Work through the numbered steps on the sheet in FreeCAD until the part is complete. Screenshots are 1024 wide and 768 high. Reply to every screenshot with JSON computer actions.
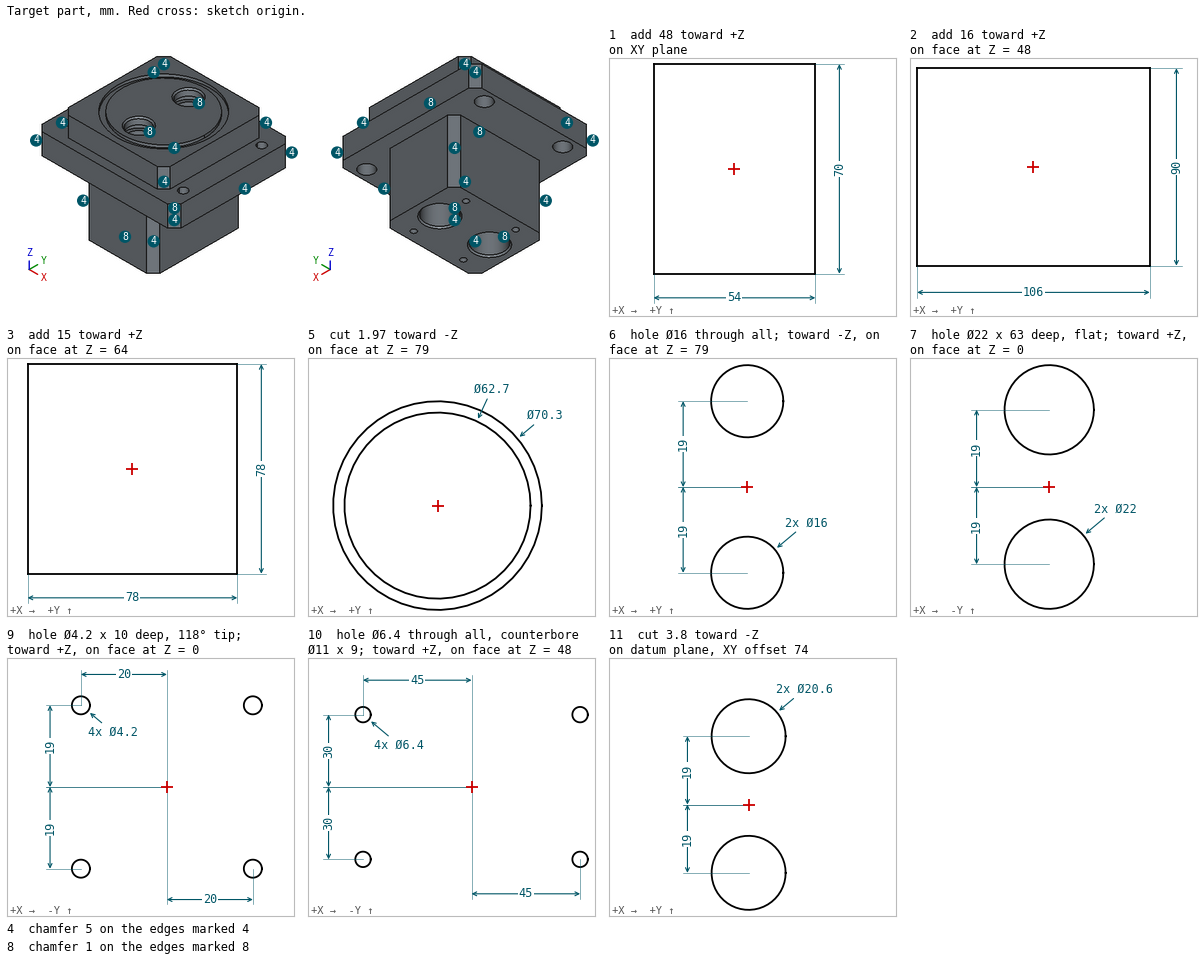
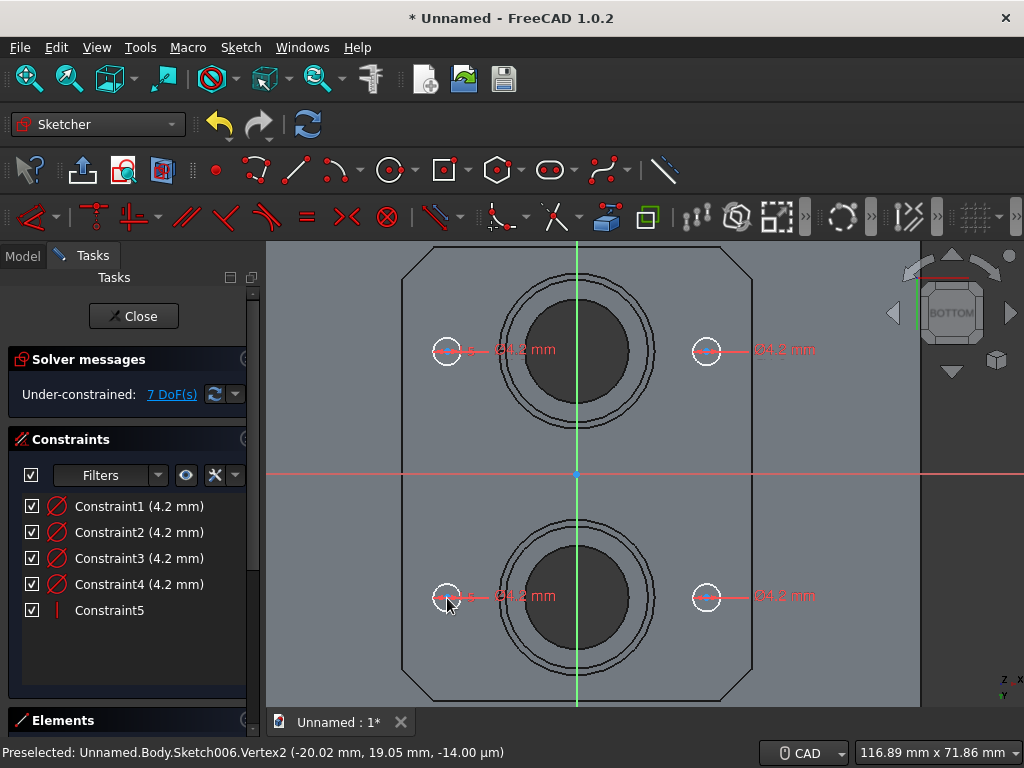
{"action": "left_click", "coordinate": [447, 598]}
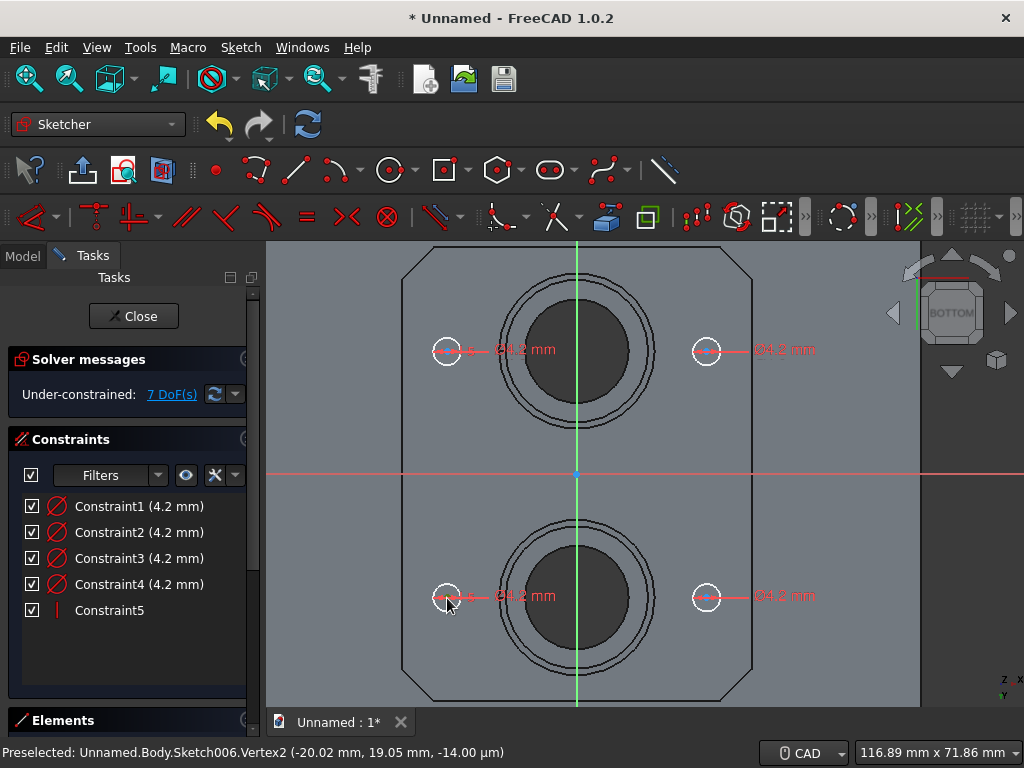
{"action": "left_click", "coordinate": [707, 598]}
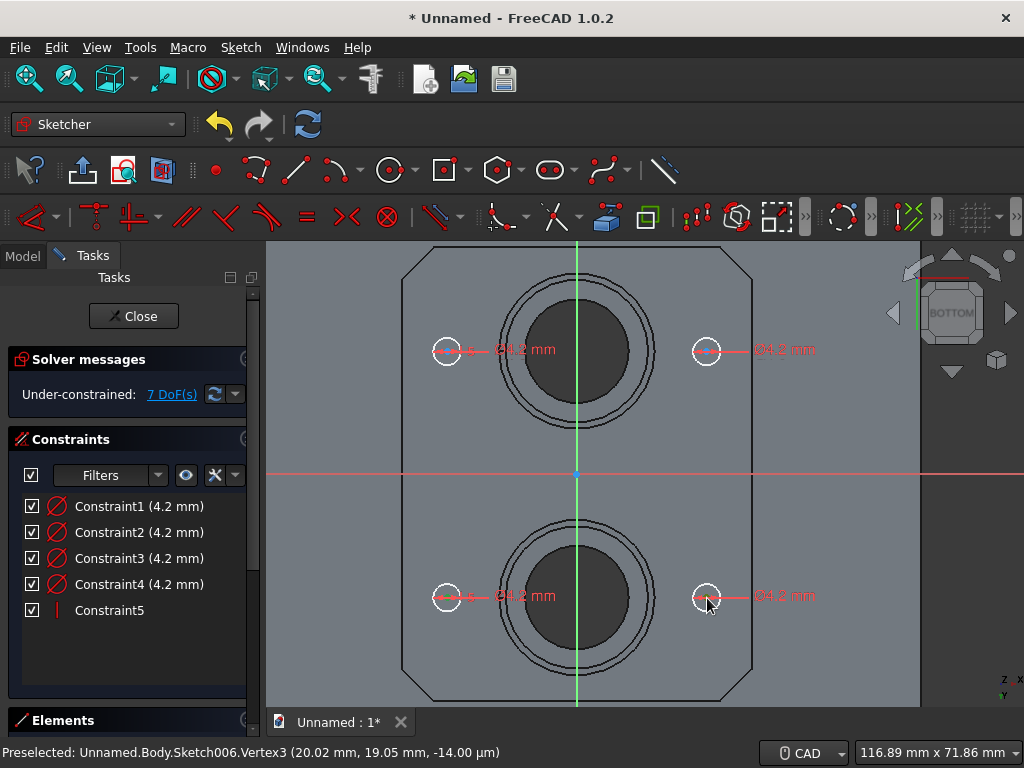
{"action": "key", "text": "h"}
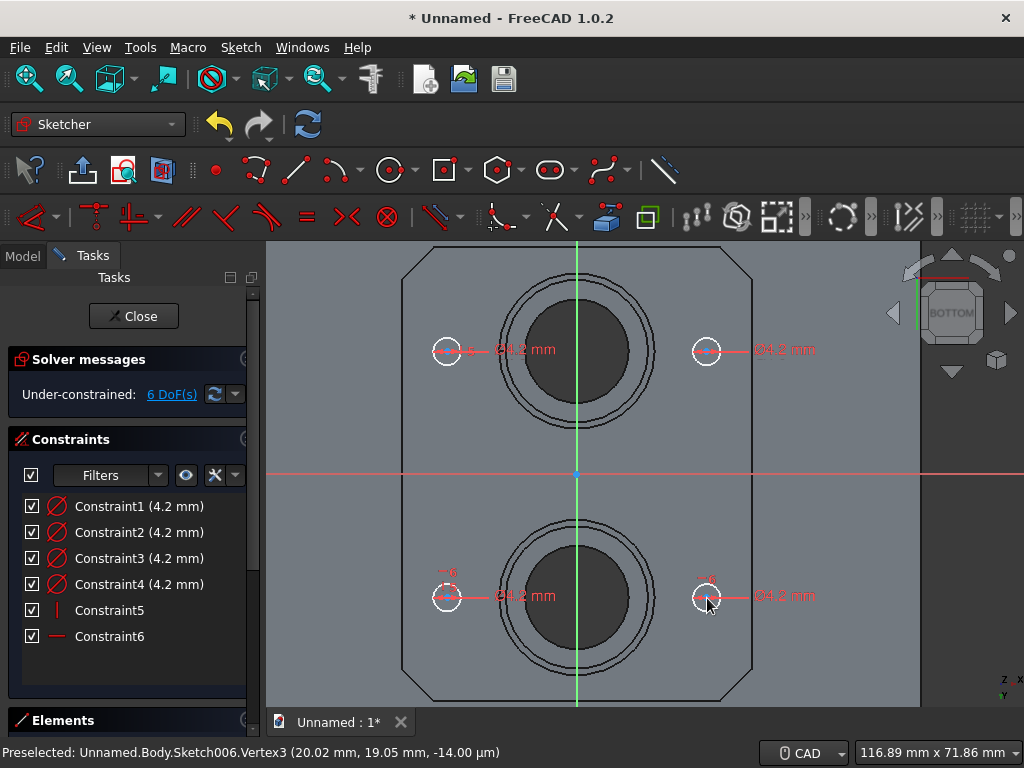
{"action": "left_click", "coordinate": [707, 598]}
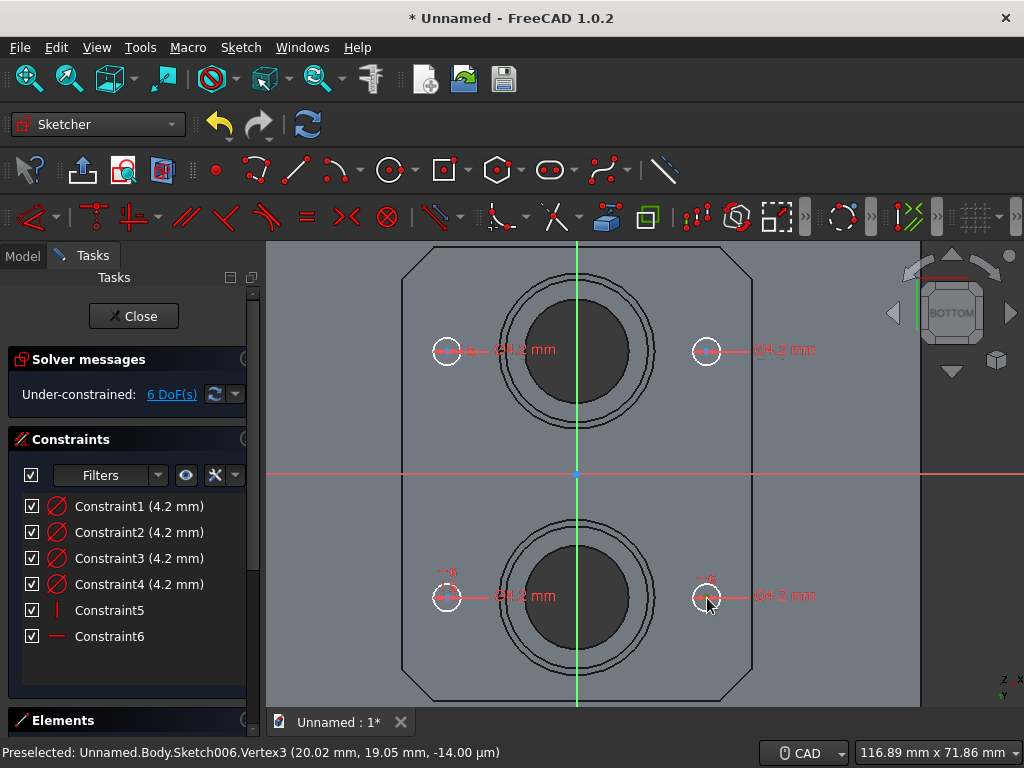
{"action": "left_click", "coordinate": [707, 352]}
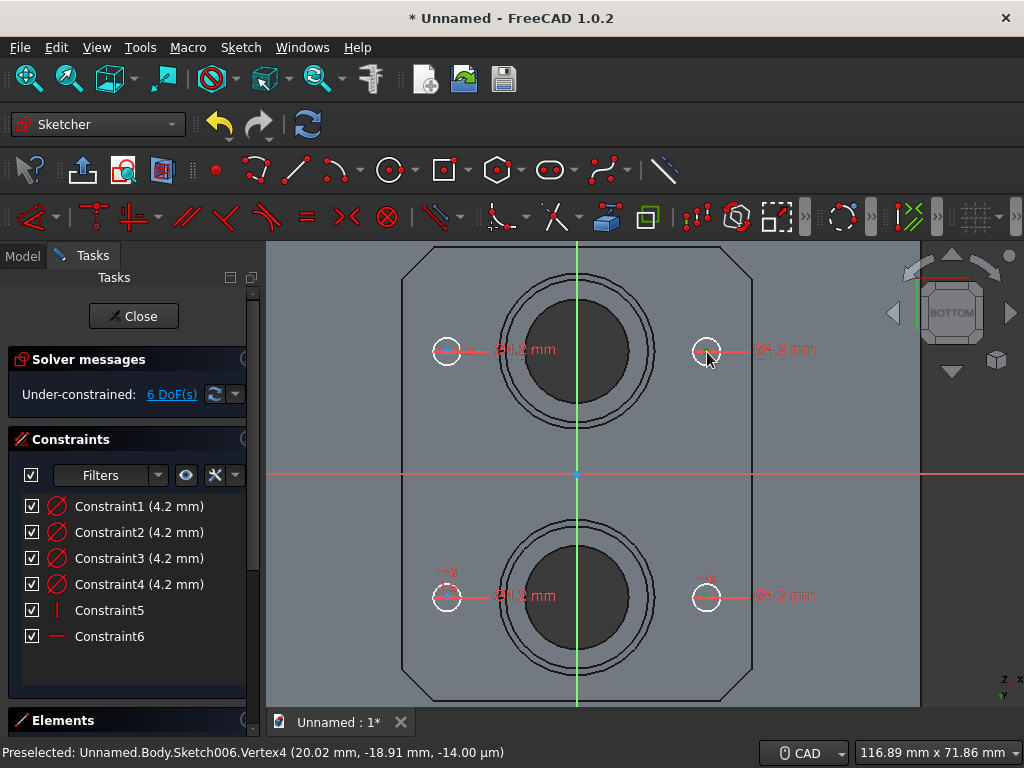
{"action": "key", "text": "v"}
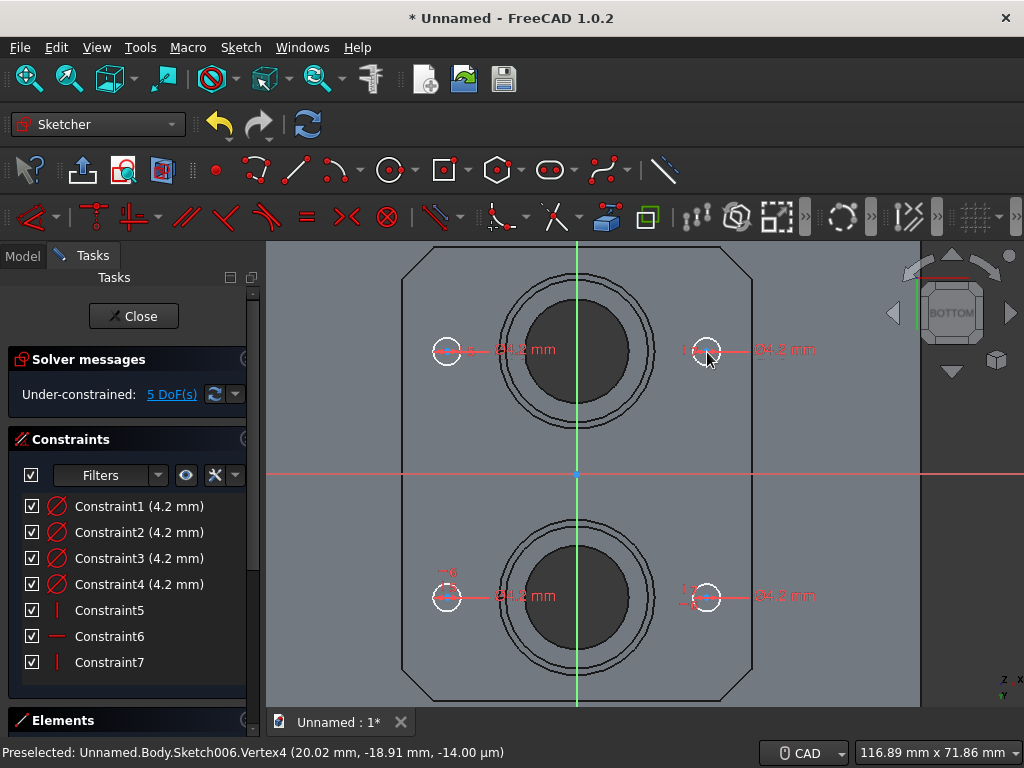
{"action": "left_click", "coordinate": [447, 352]}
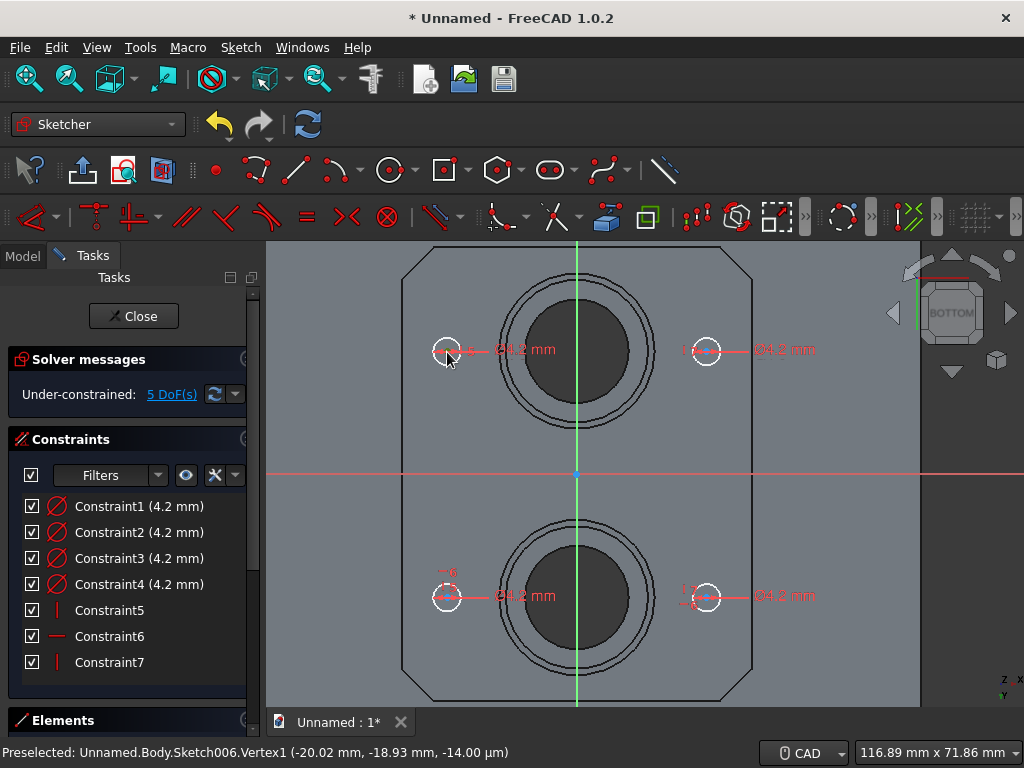
{"action": "left_click", "coordinate": [707, 352]}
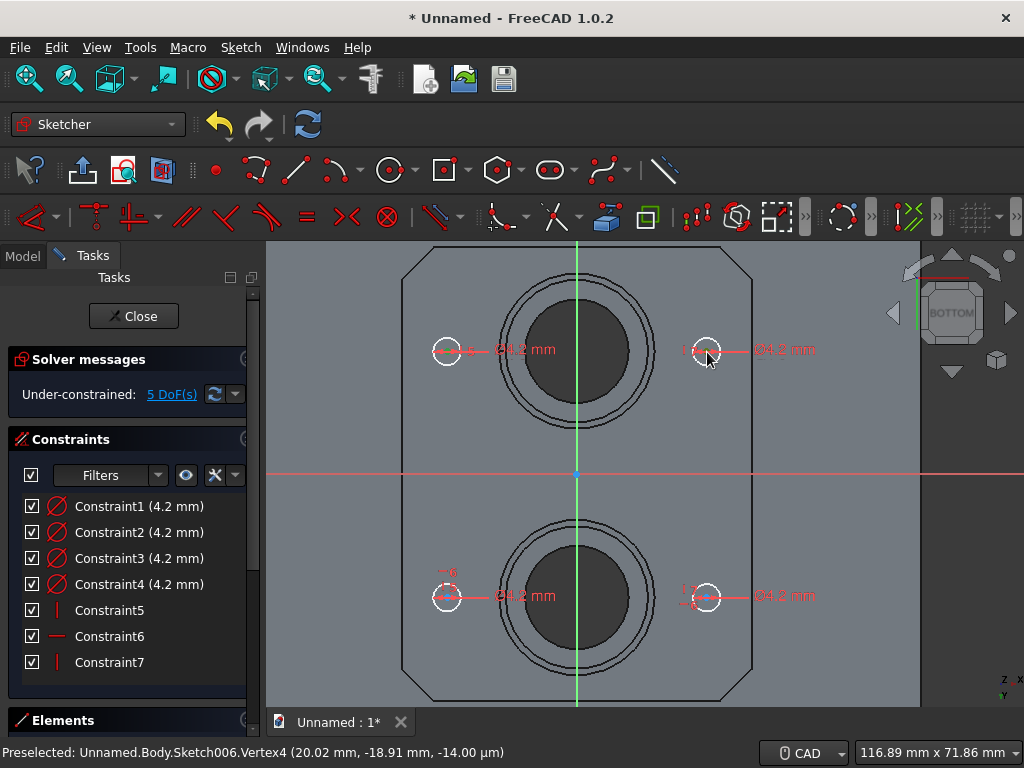
{"action": "left_click", "coordinate": [160, 218]}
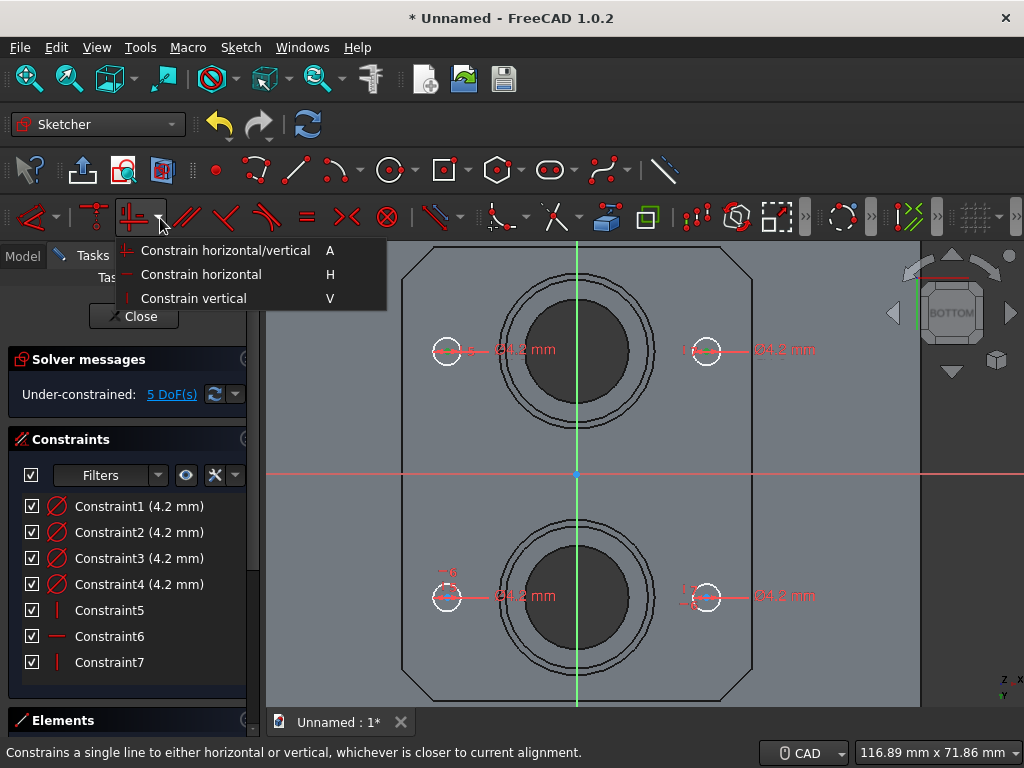
{"action": "left_click", "coordinate": [251, 274]}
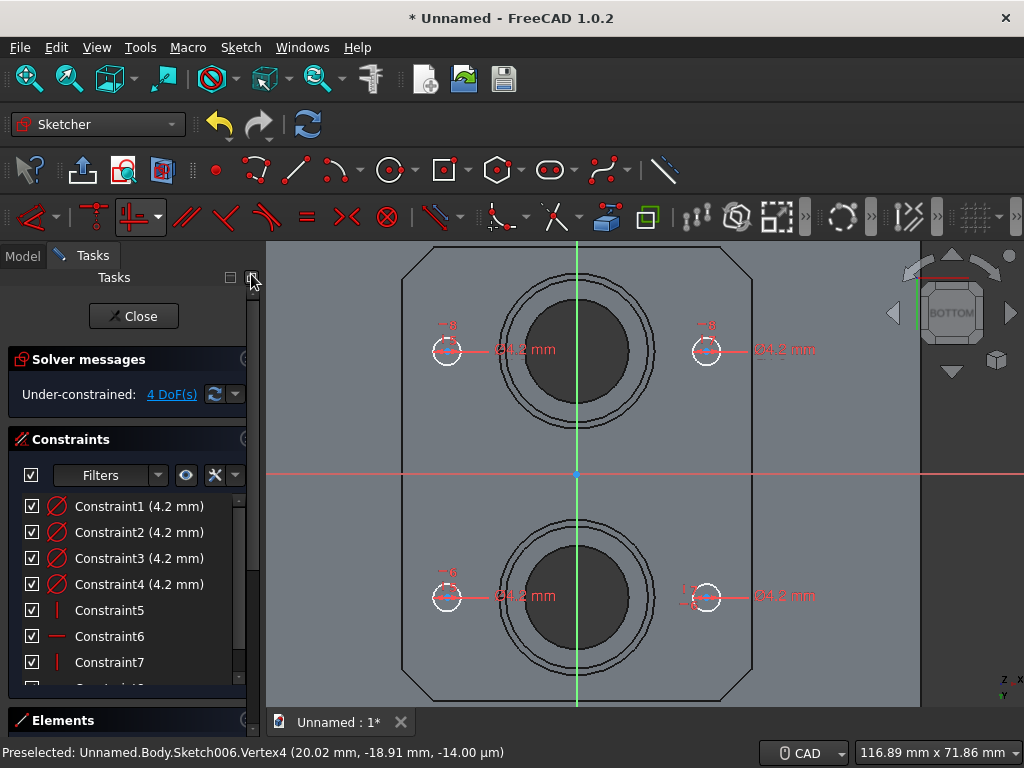
{"action": "left_click", "coordinate": [32, 218]}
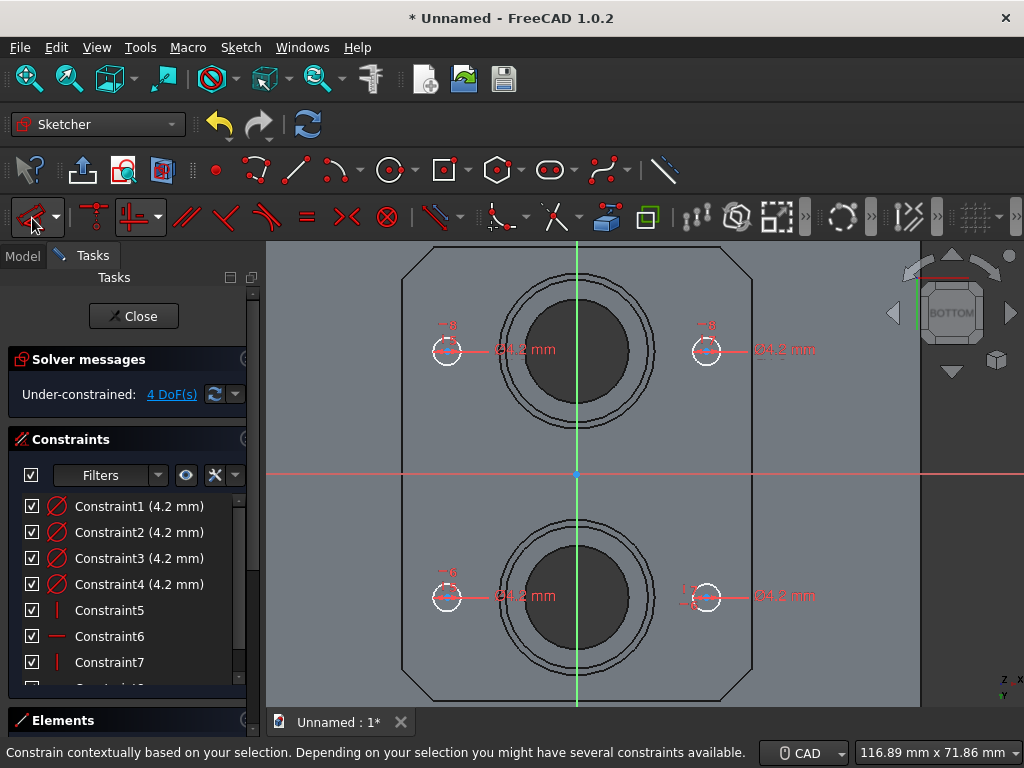
{"action": "left_click", "coordinate": [447, 352]}
{"action": "left_click", "coordinate": [512, 318]}